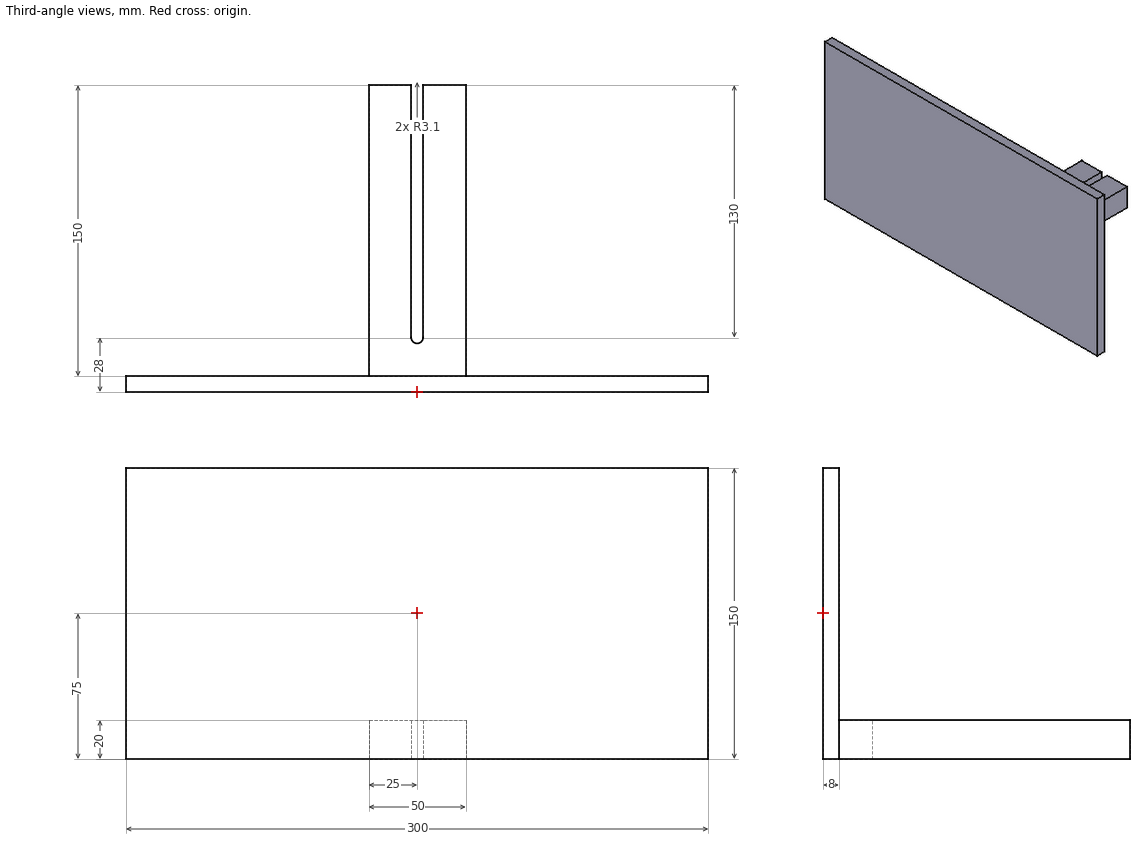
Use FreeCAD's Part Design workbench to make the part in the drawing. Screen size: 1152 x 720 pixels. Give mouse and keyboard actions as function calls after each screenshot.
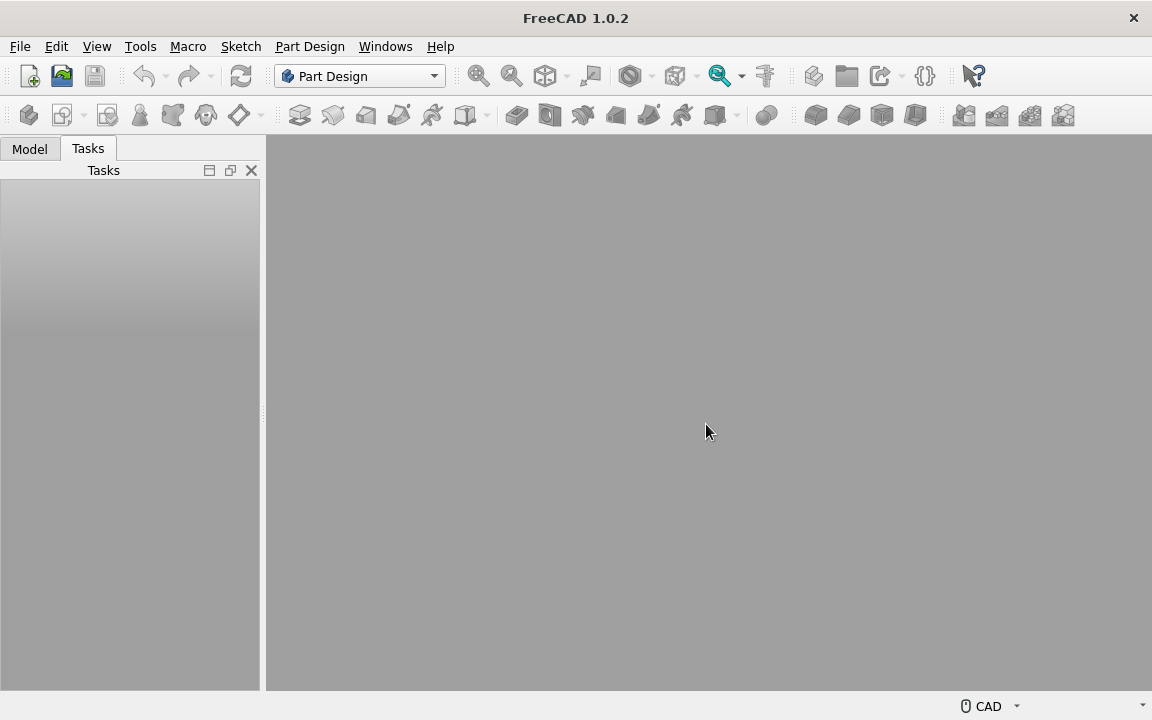
click(29, 76)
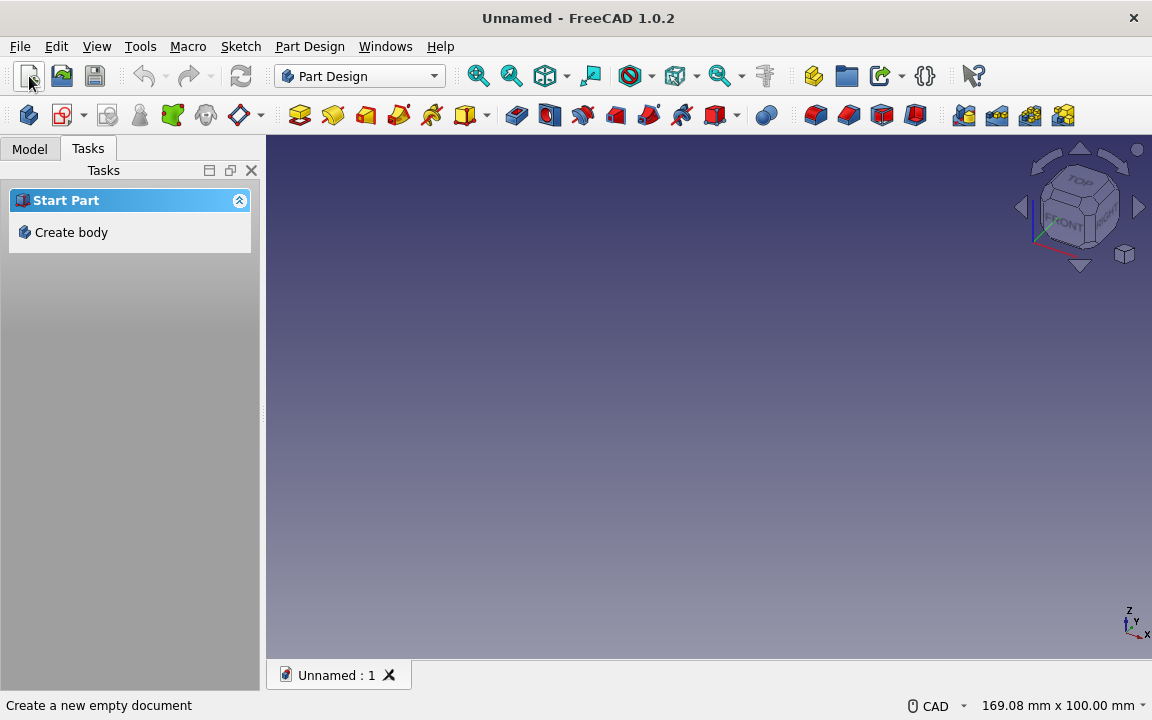
click(62, 116)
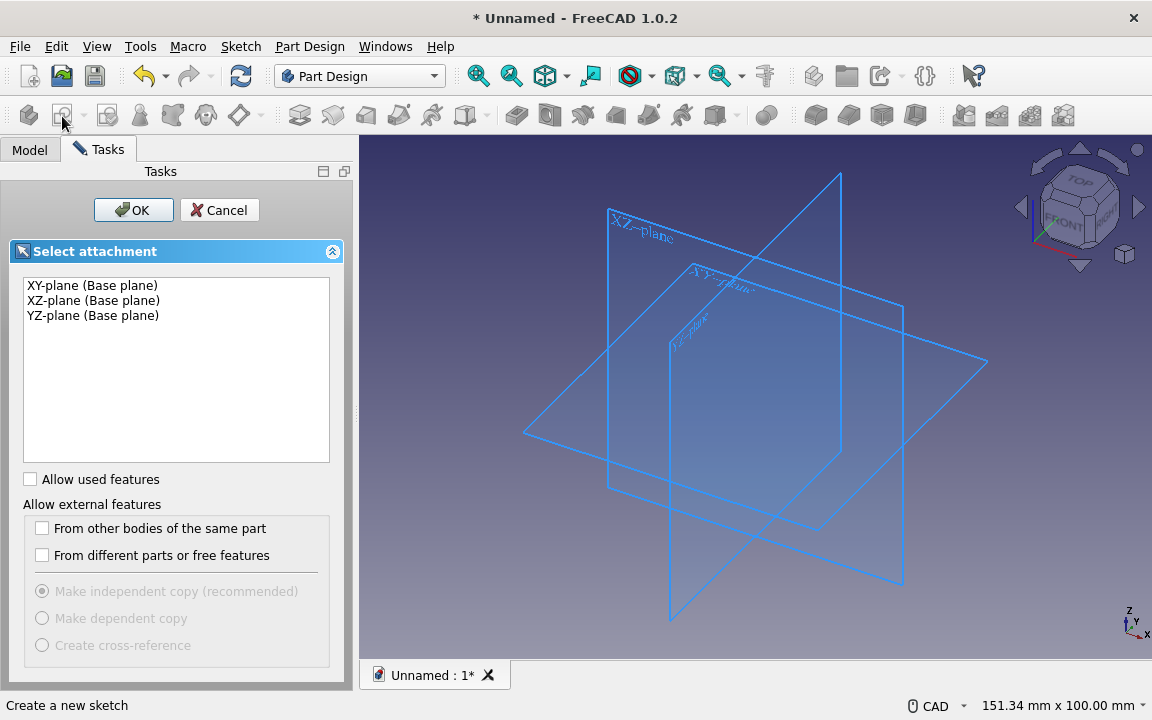
click(84, 300)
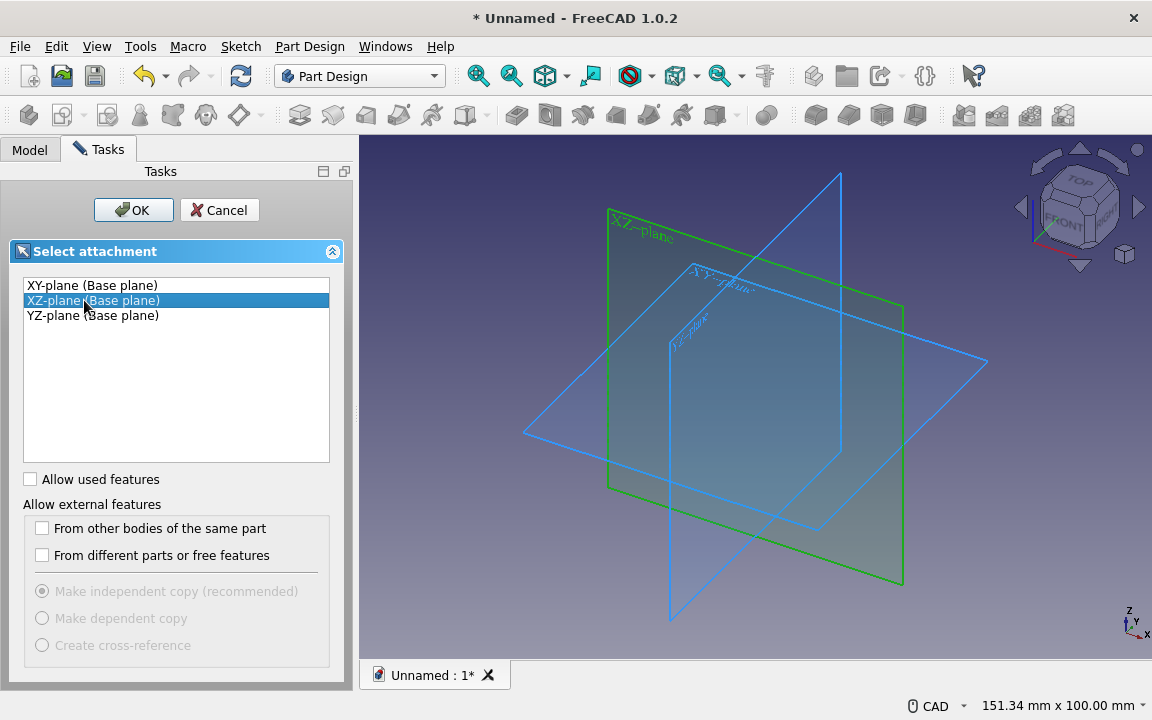
click(134, 210)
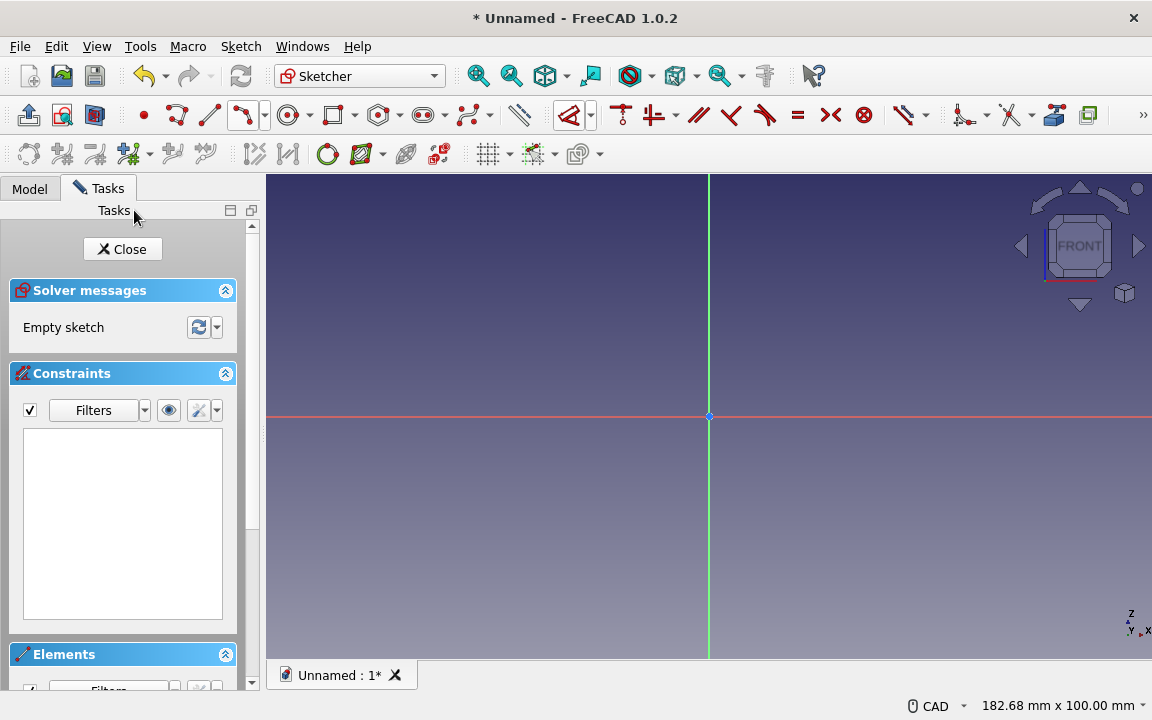
scroll(601, 417, down, 5)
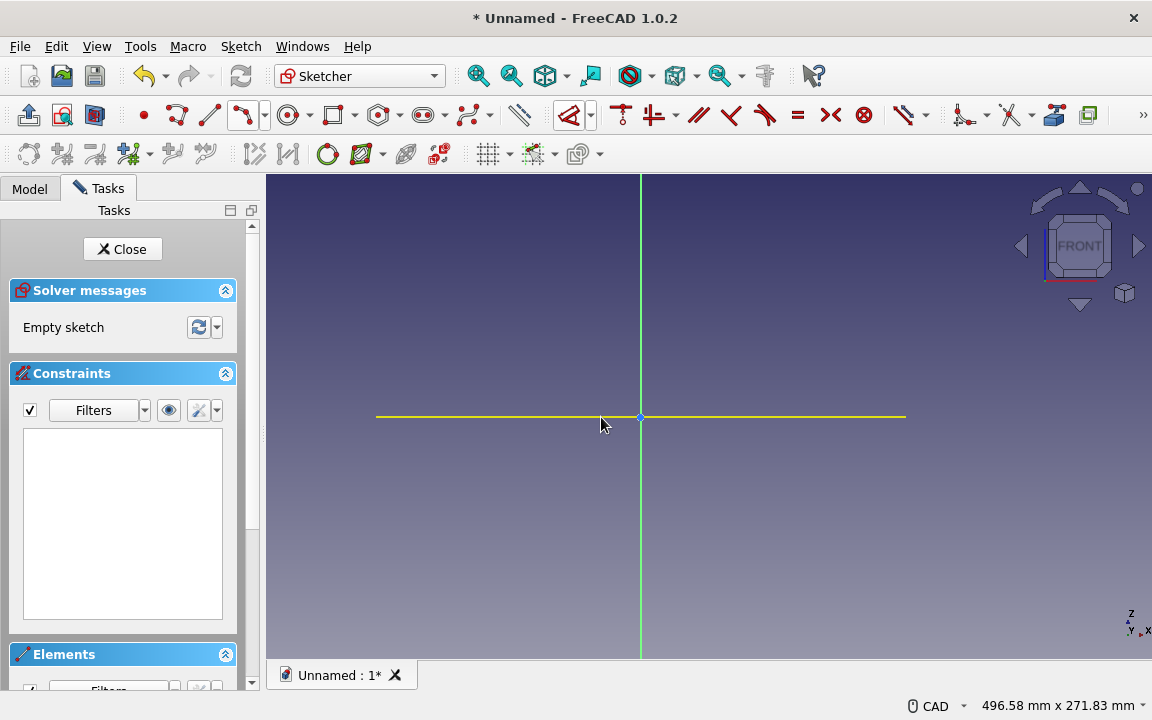
click(354, 116)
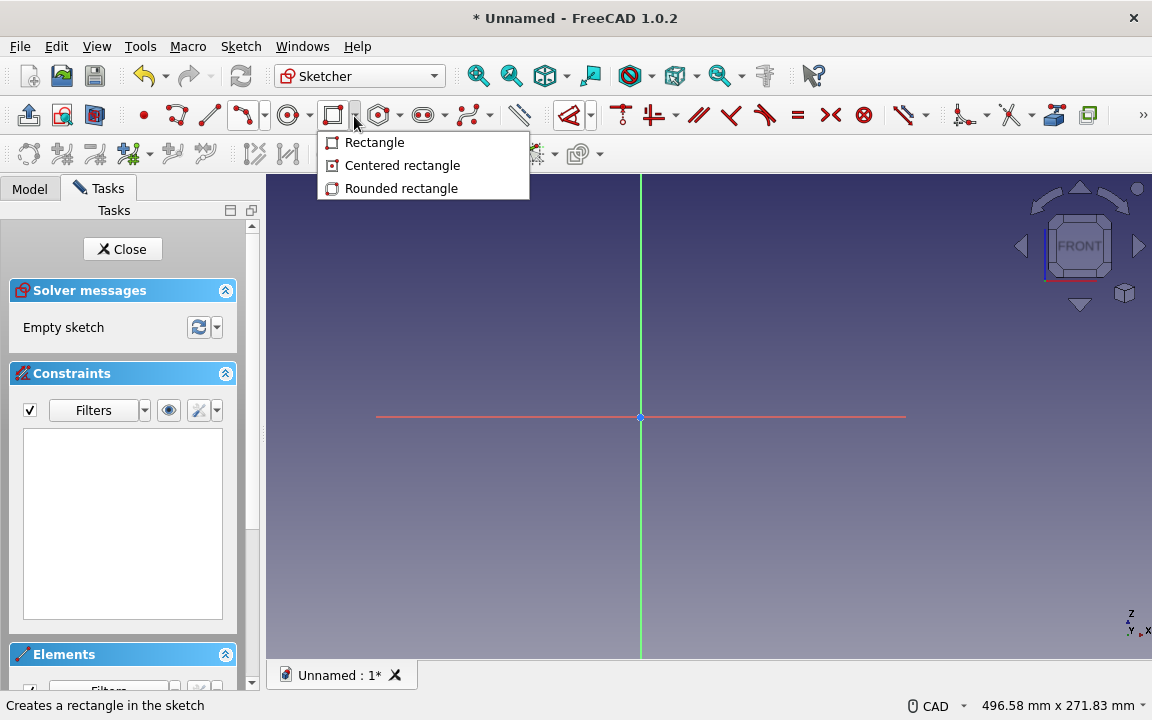
click(424, 166)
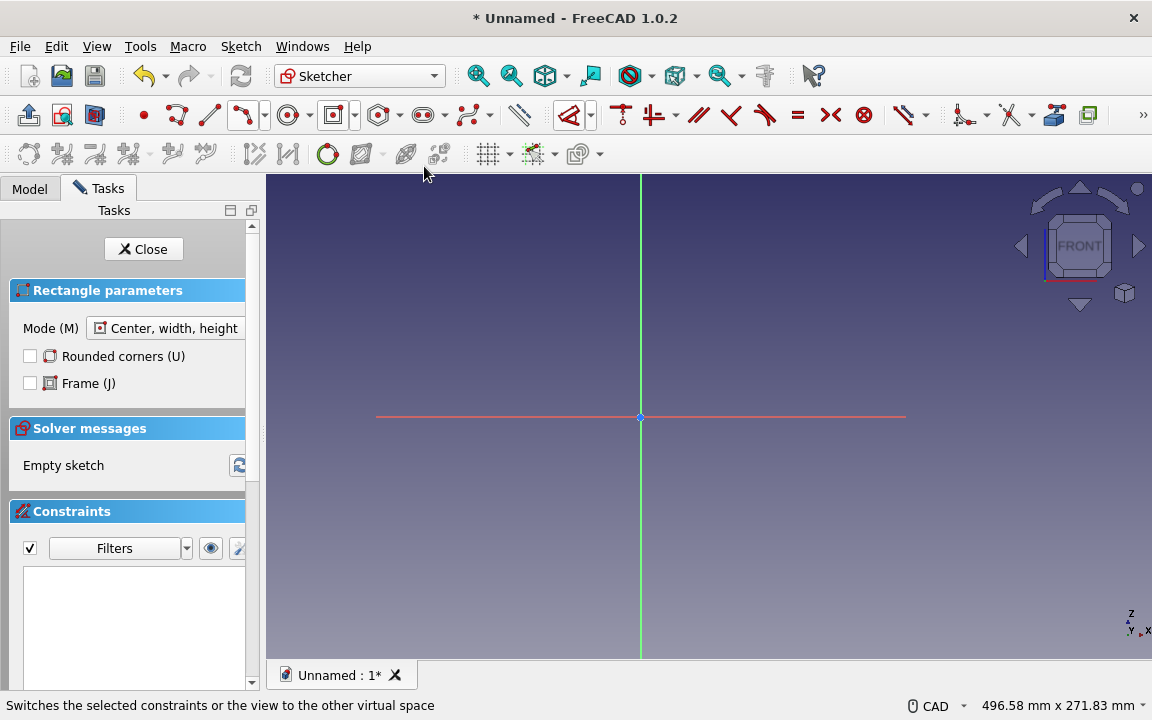
click(641, 417)
click(909, 283)
key(Escape)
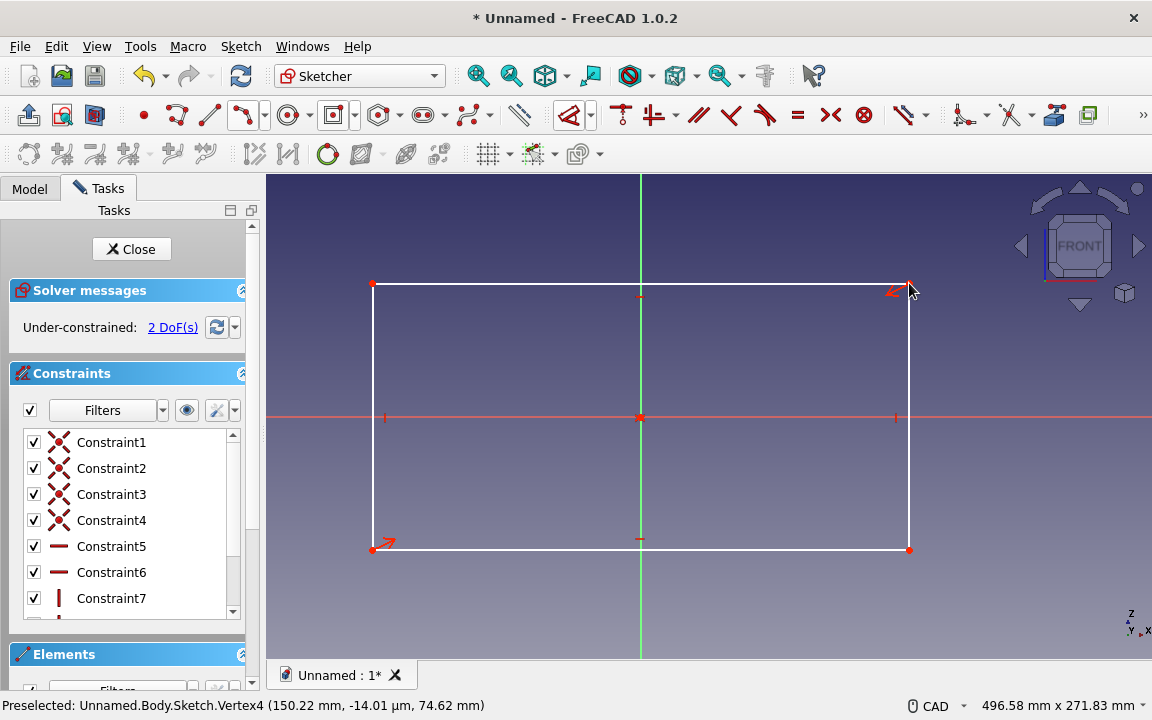
click(568, 116)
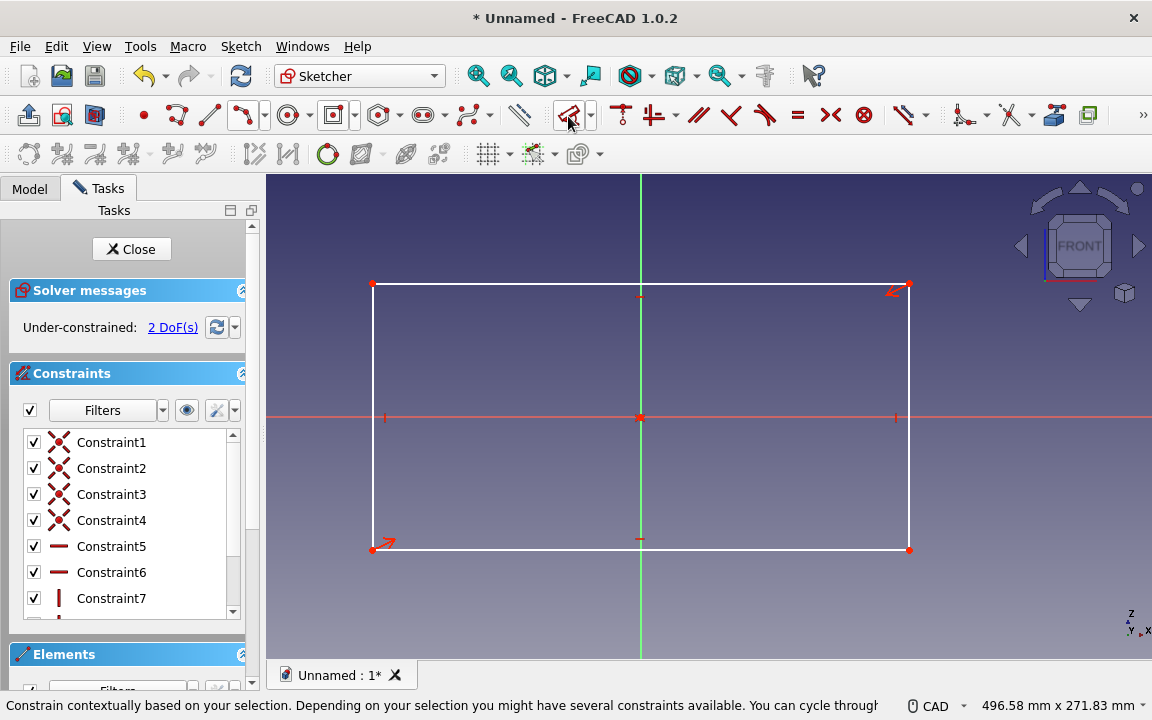
click(534, 550)
click(518, 584)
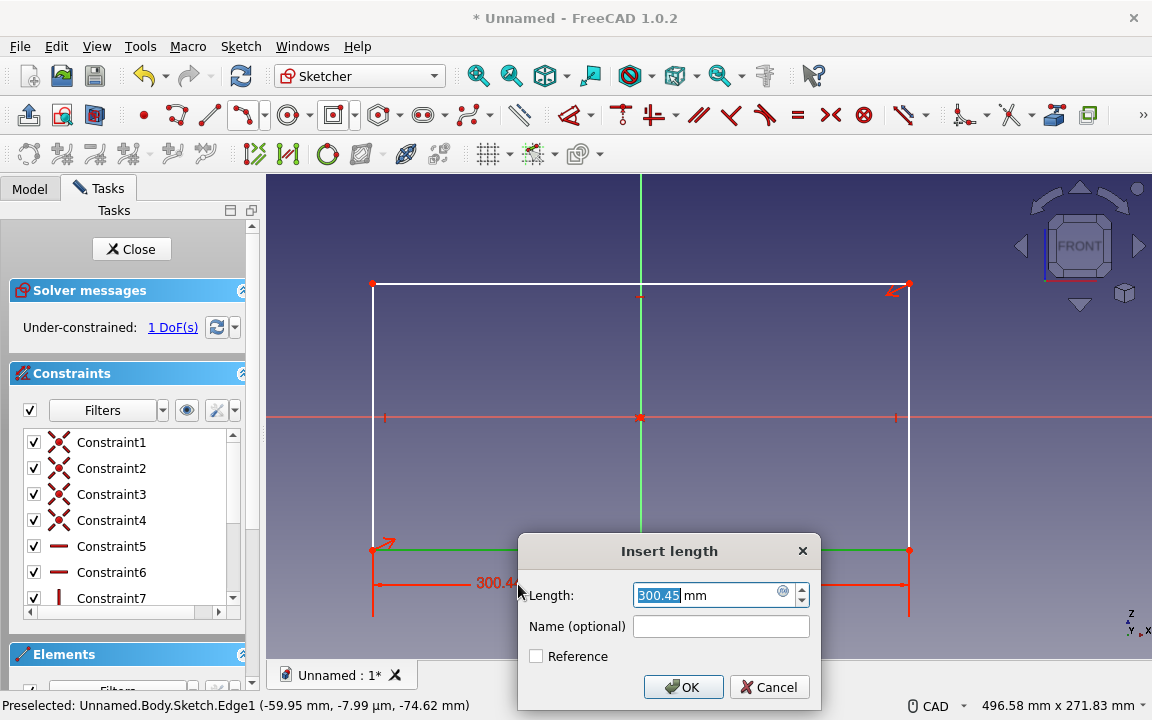
text(300)
key(Return)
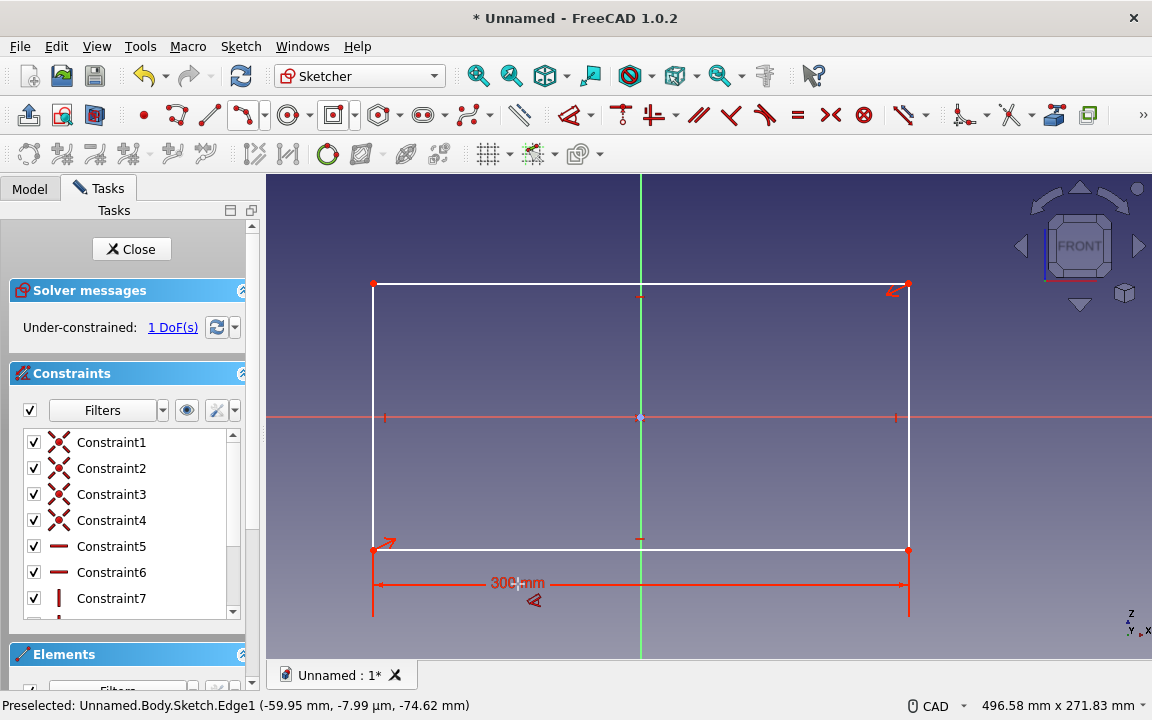
click(909, 470)
click(943, 356)